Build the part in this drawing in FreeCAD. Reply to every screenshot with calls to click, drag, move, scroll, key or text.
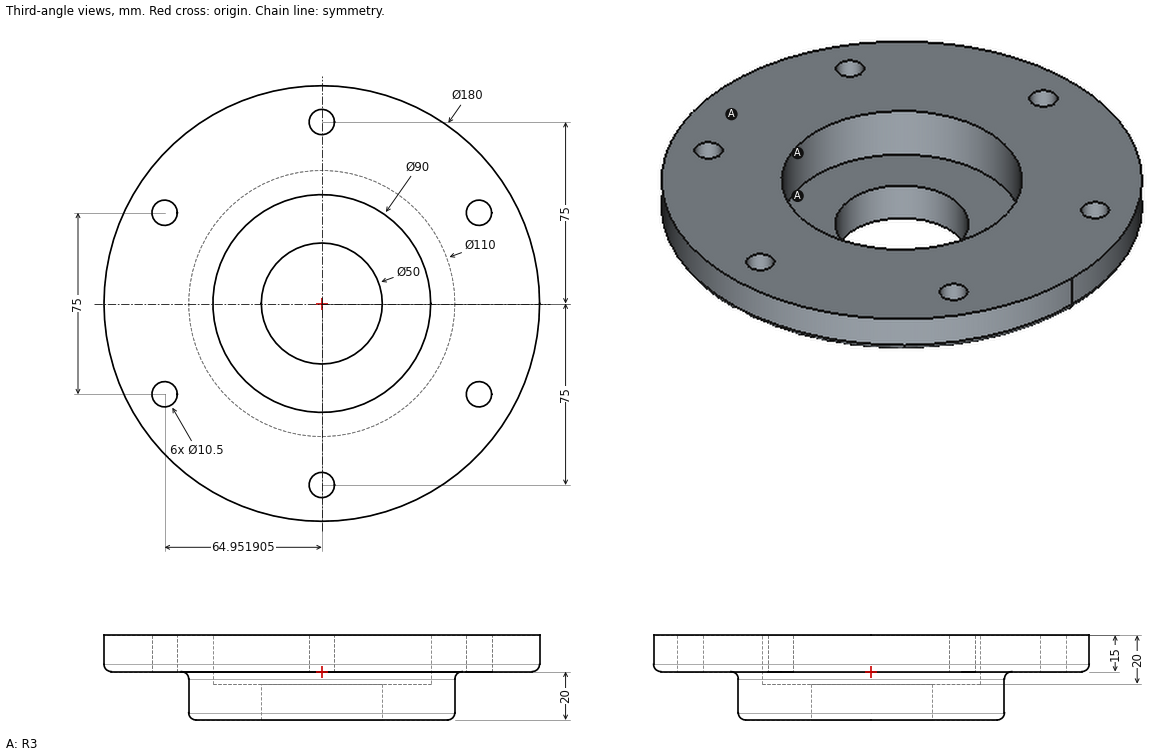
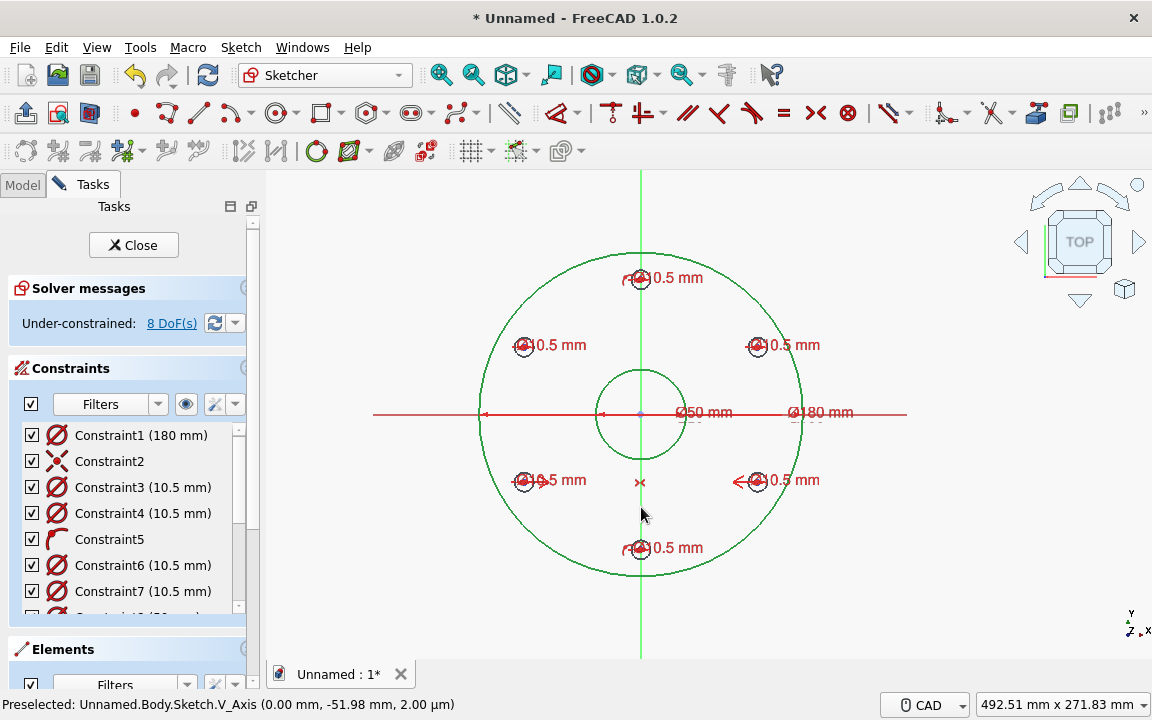
click(524, 482)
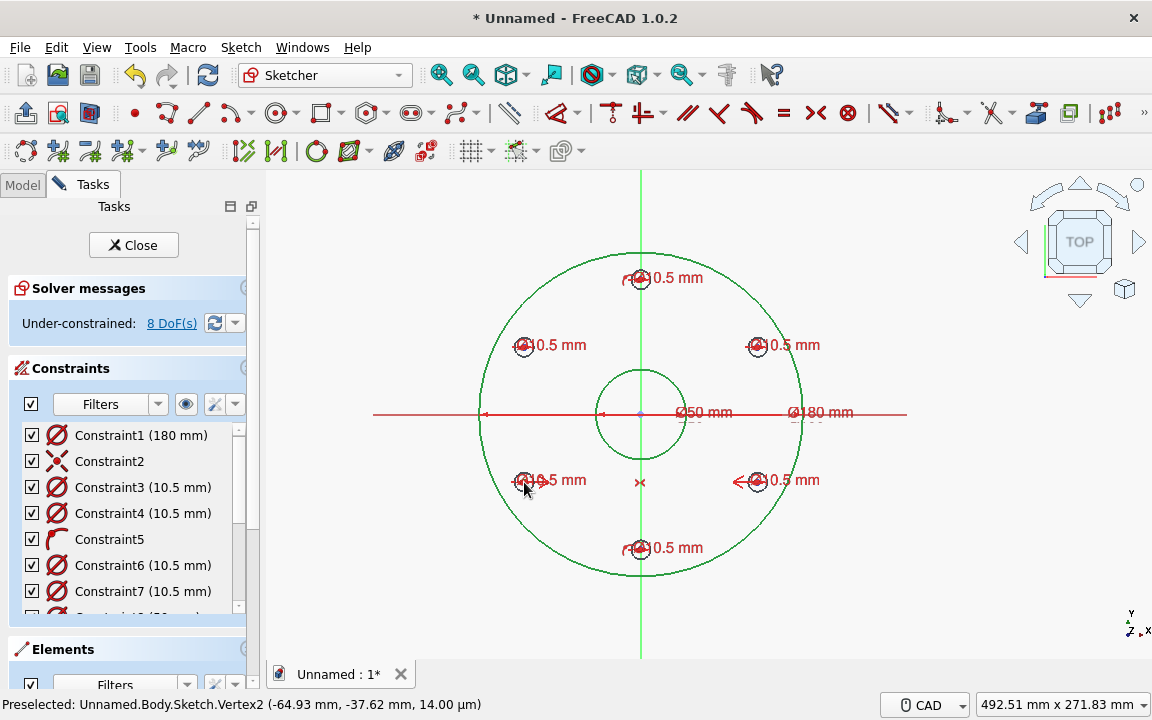
click(524, 347)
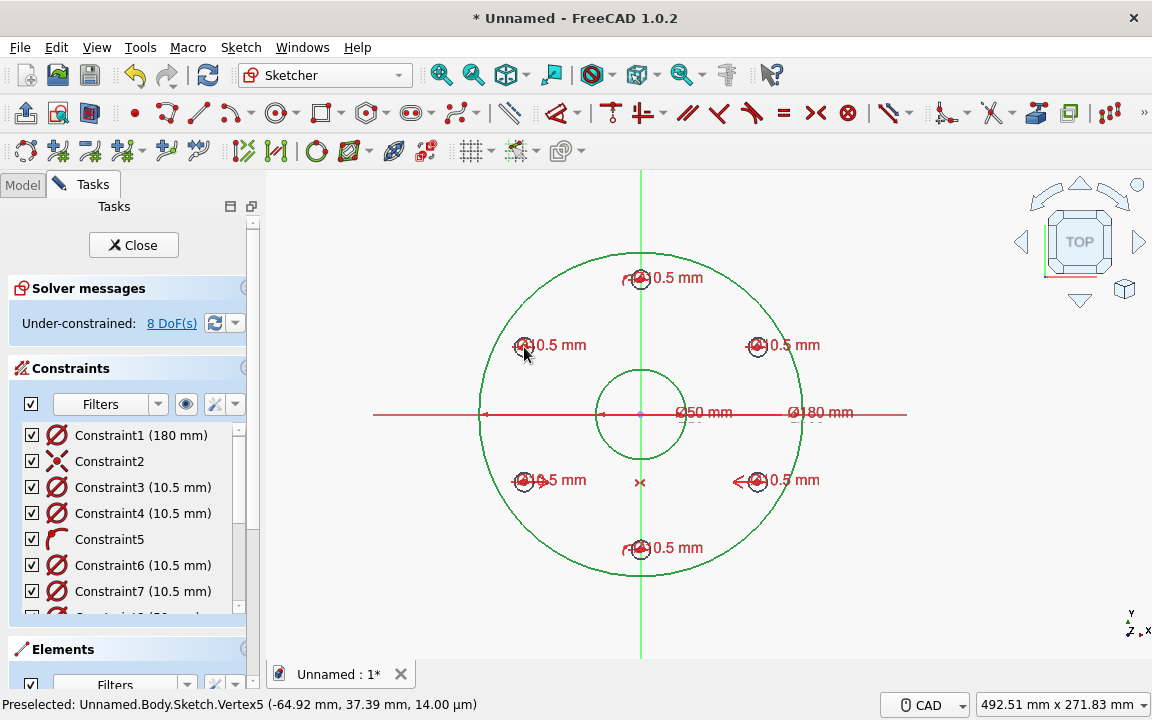
click(393, 414)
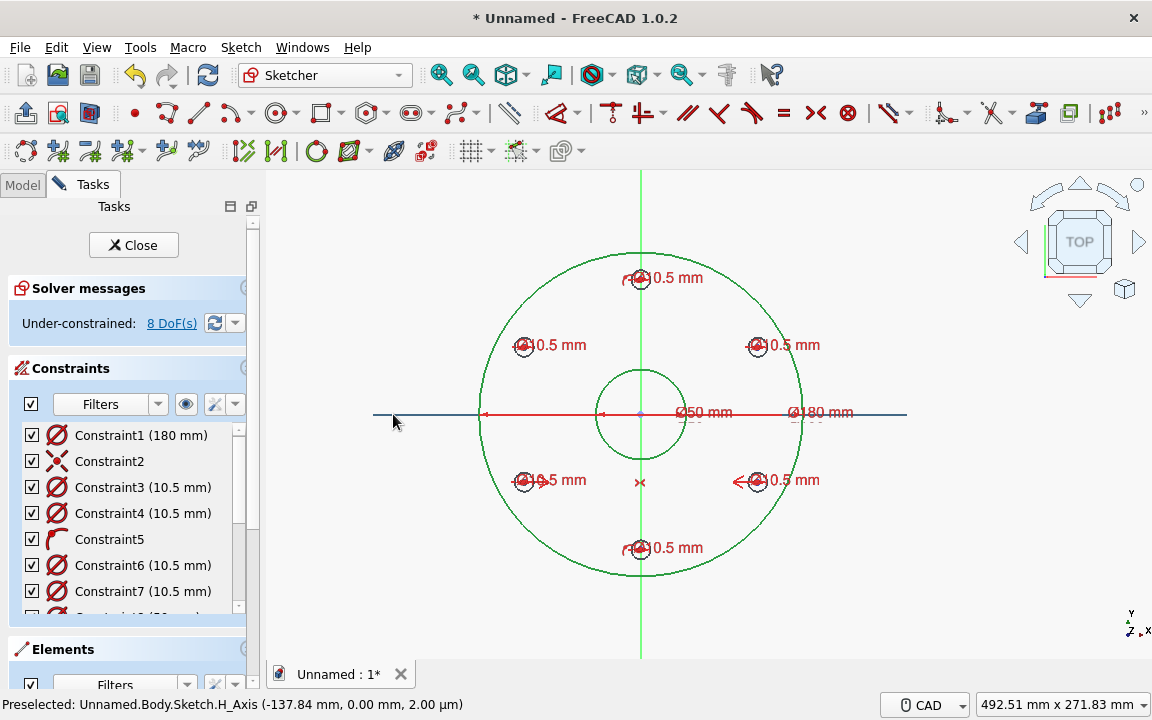
click(816, 114)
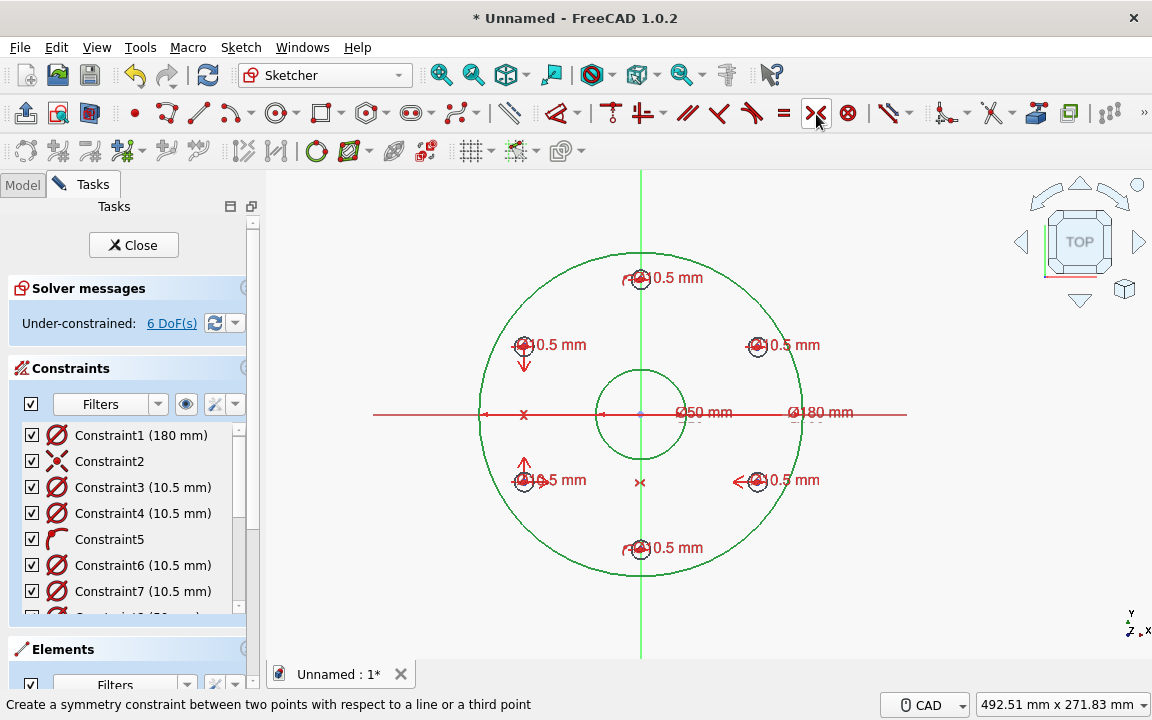
click(758, 482)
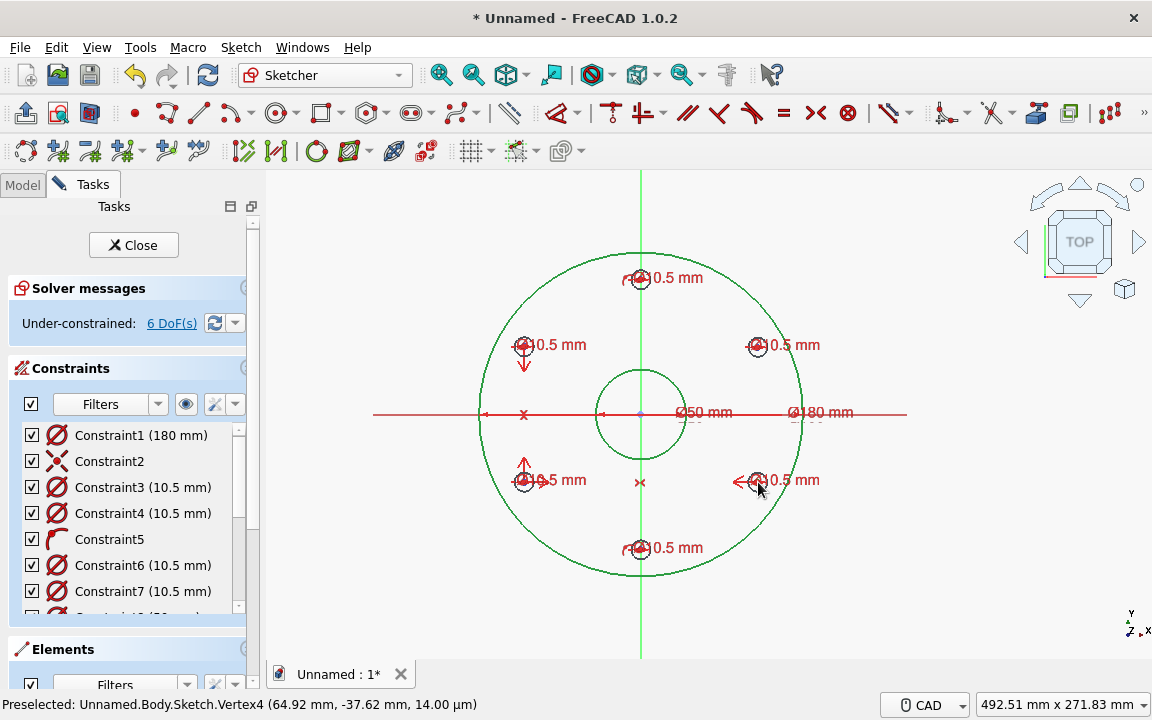
click(758, 347)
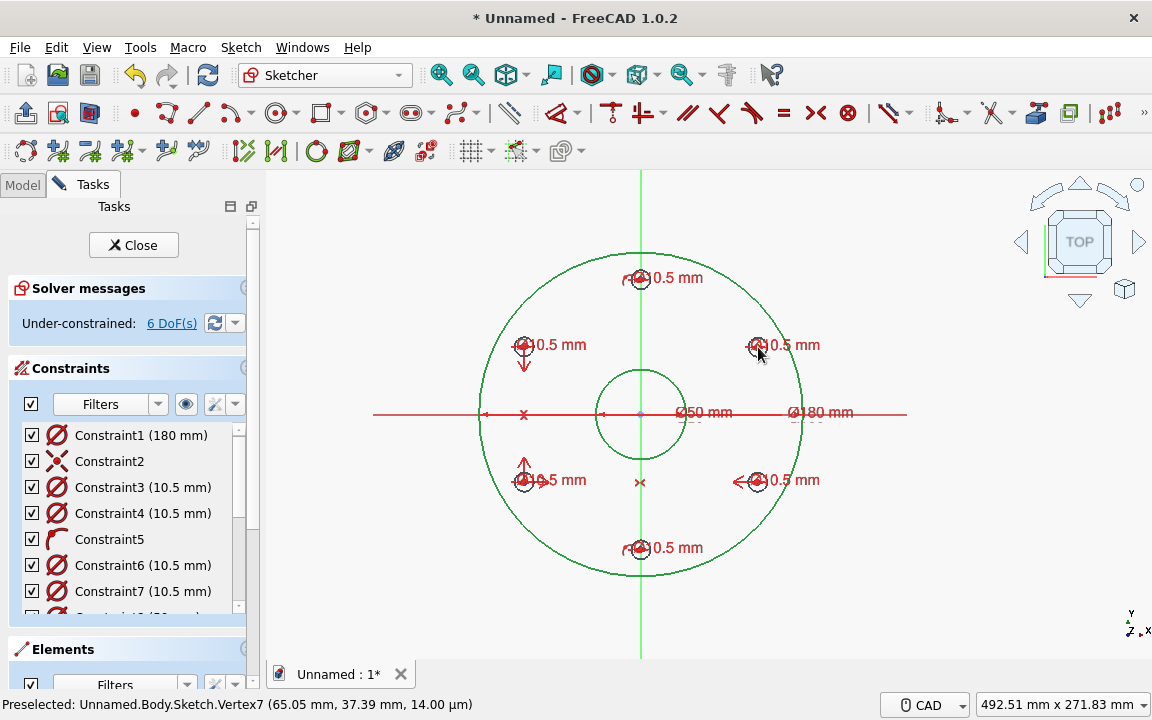
click(393, 414)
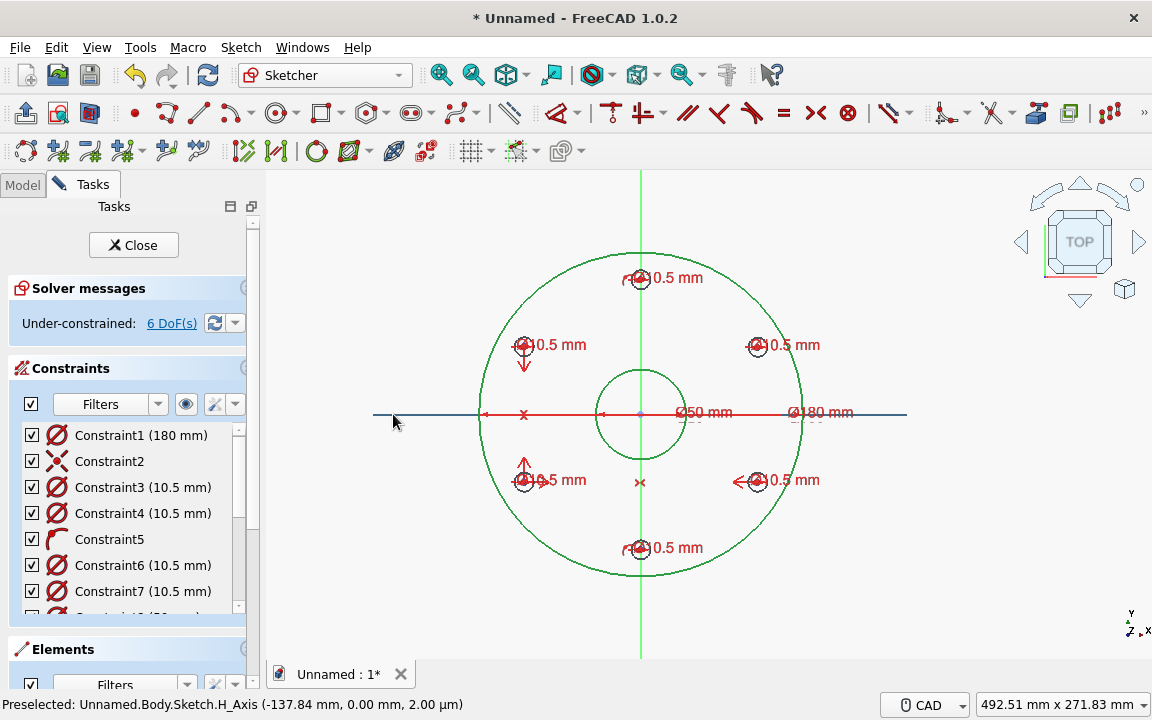
key(s)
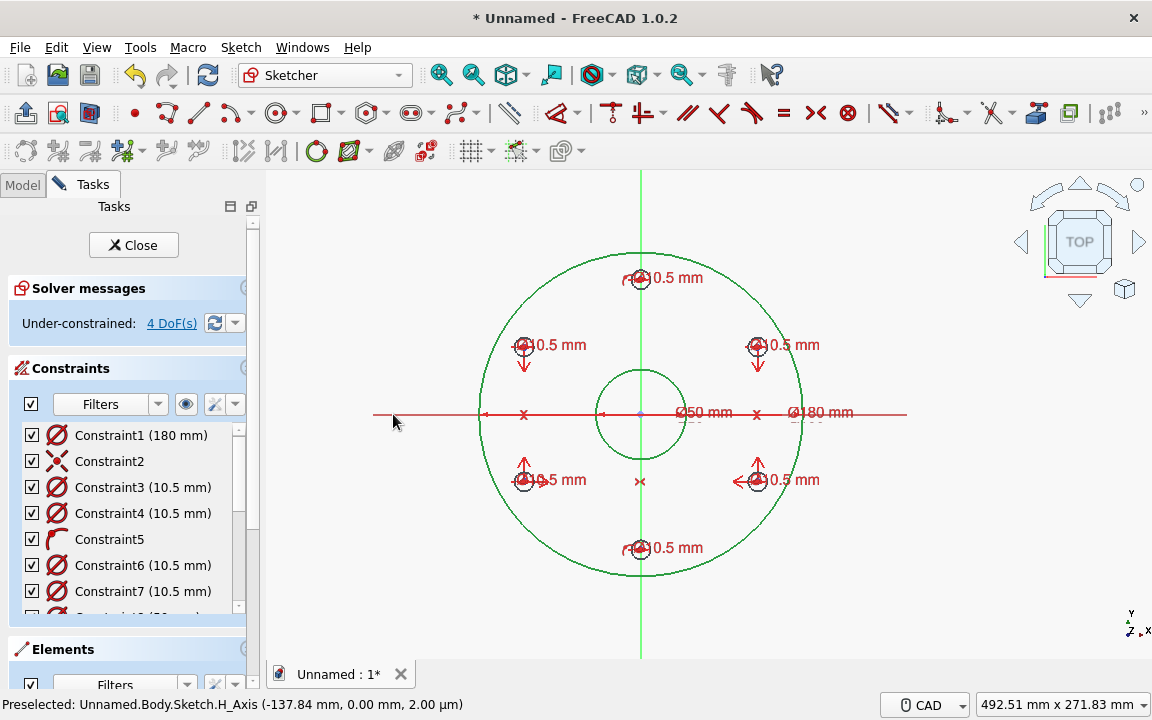
key(d)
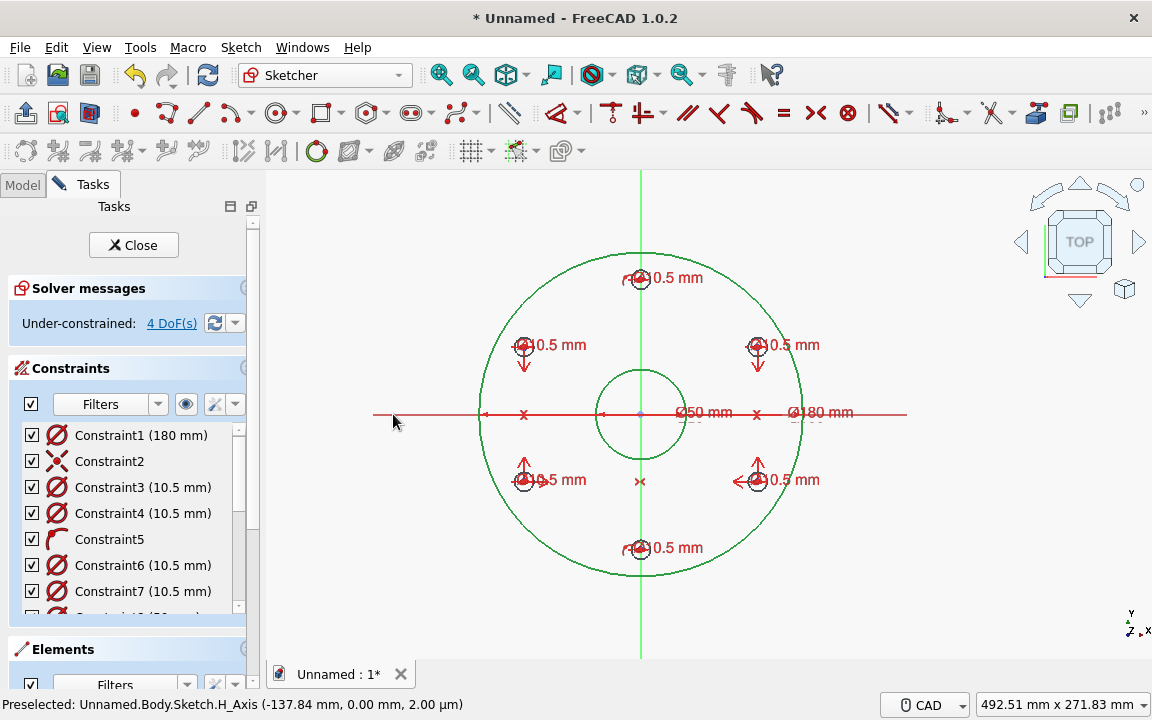
click(641, 550)
click(675, 482)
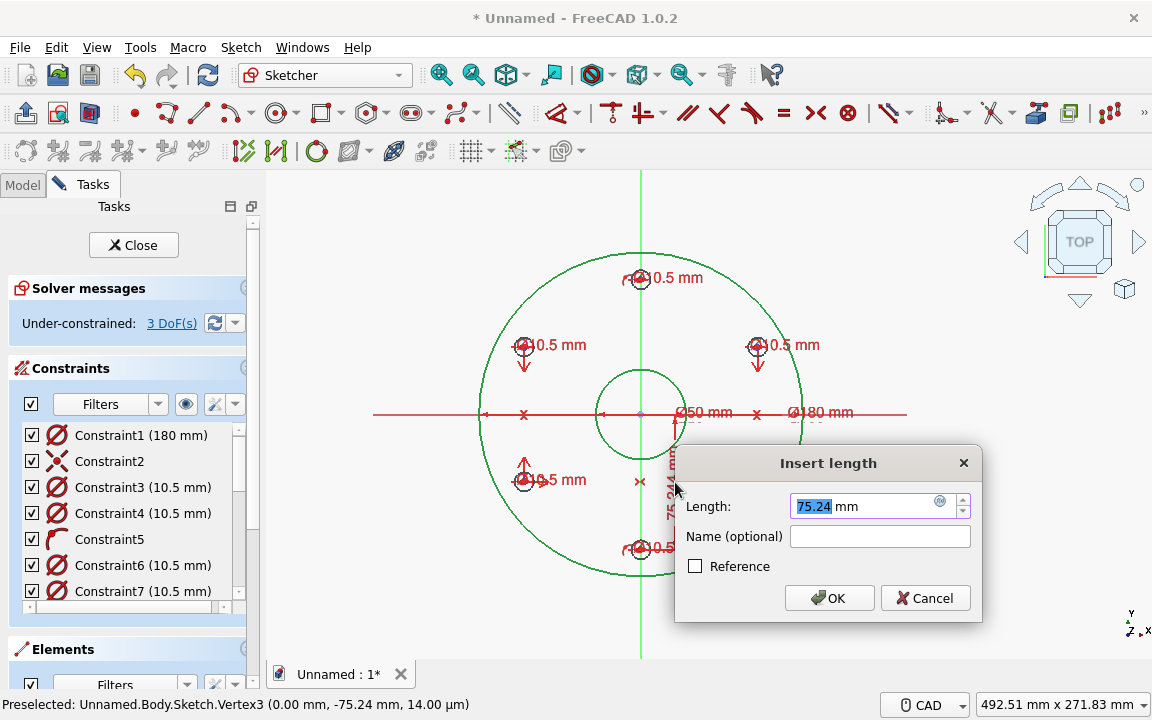
text(75)
key(Return)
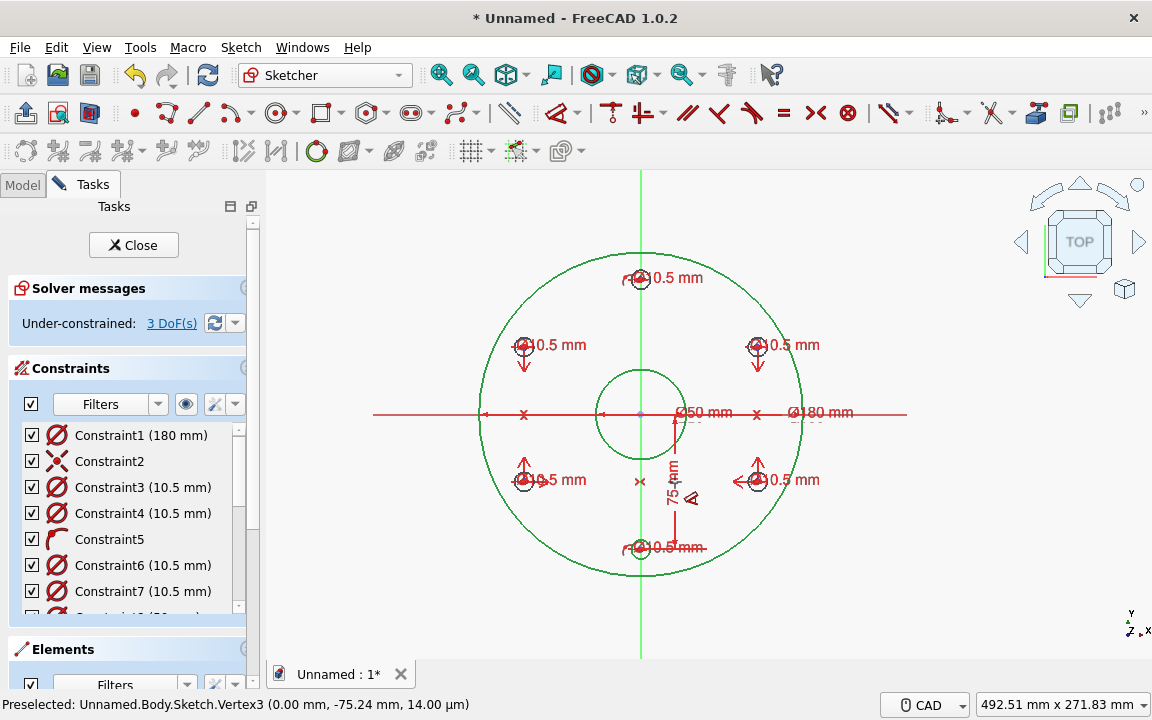
click(641, 280)
click(675, 347)